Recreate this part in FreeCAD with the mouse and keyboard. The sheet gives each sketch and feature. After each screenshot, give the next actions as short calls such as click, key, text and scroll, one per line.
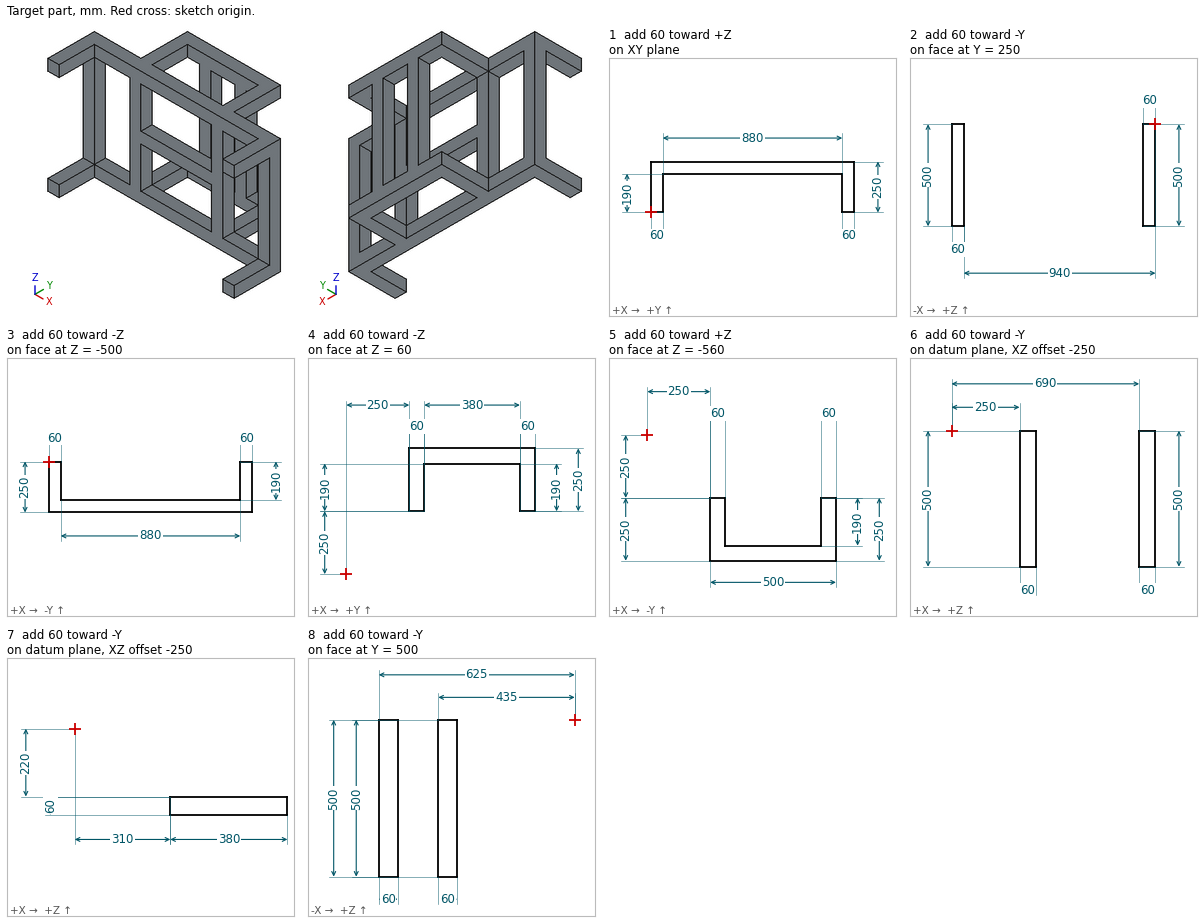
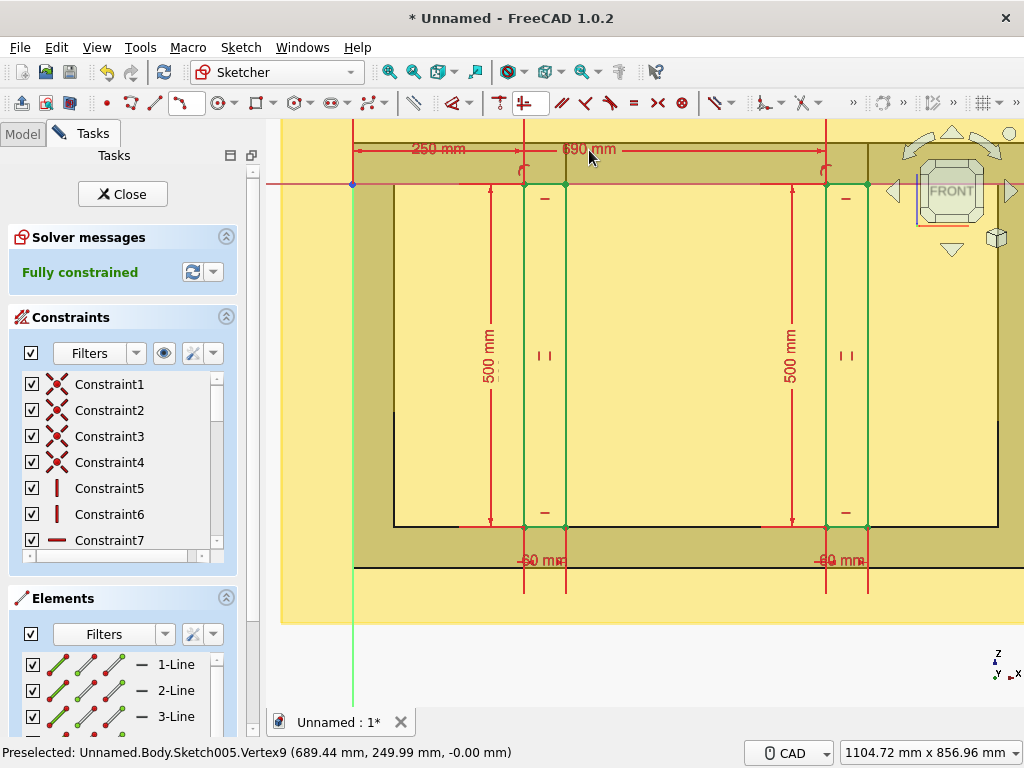
click(123, 194)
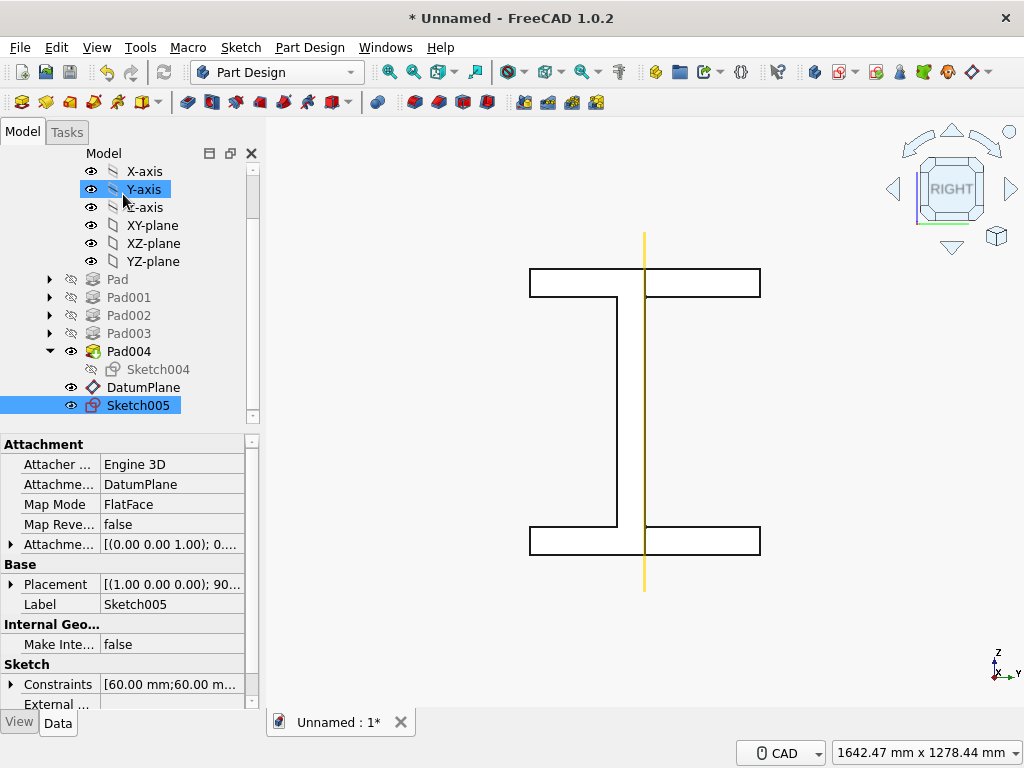
click(22, 102)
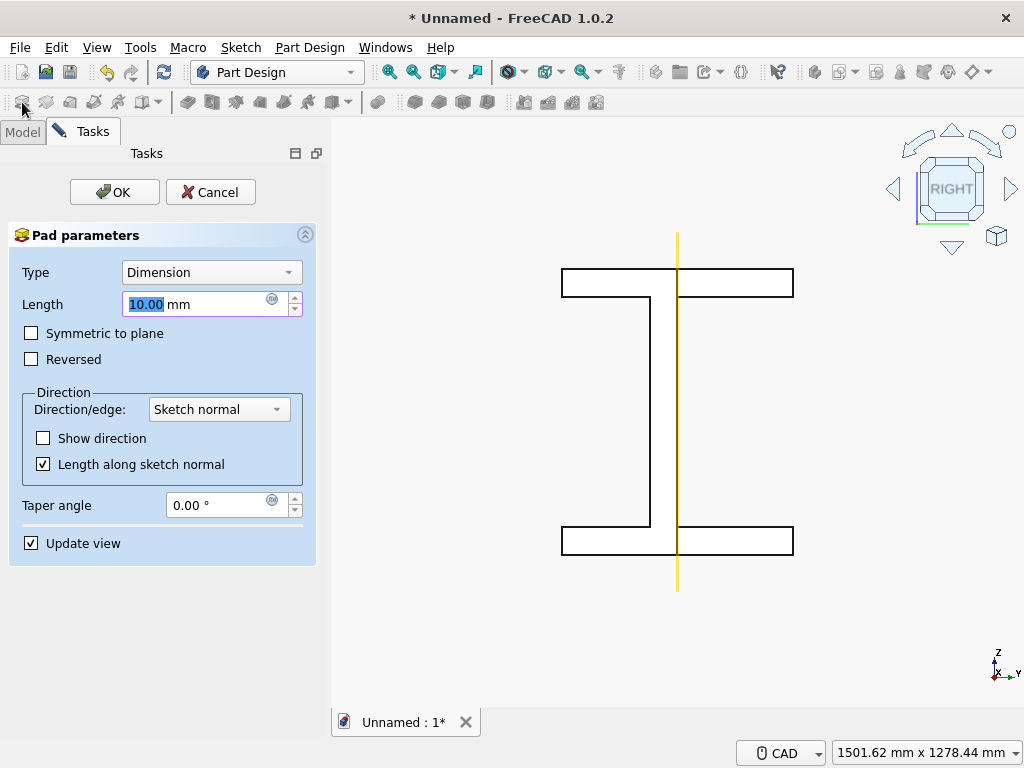
text(60)
key(Tab)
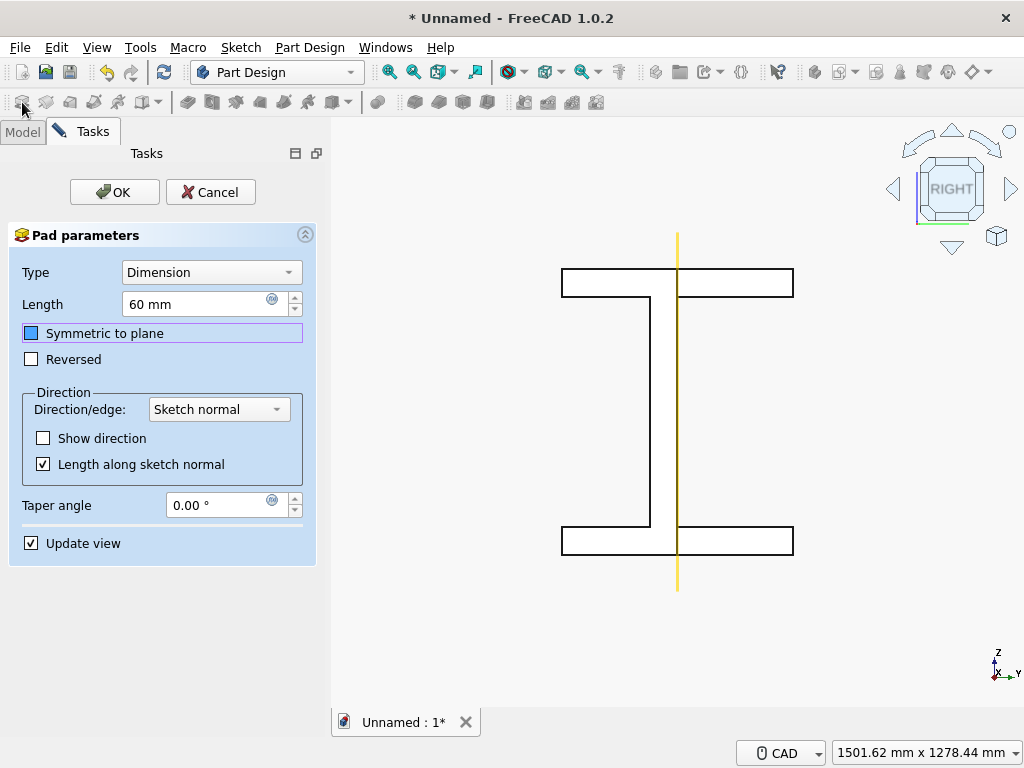
click(115, 192)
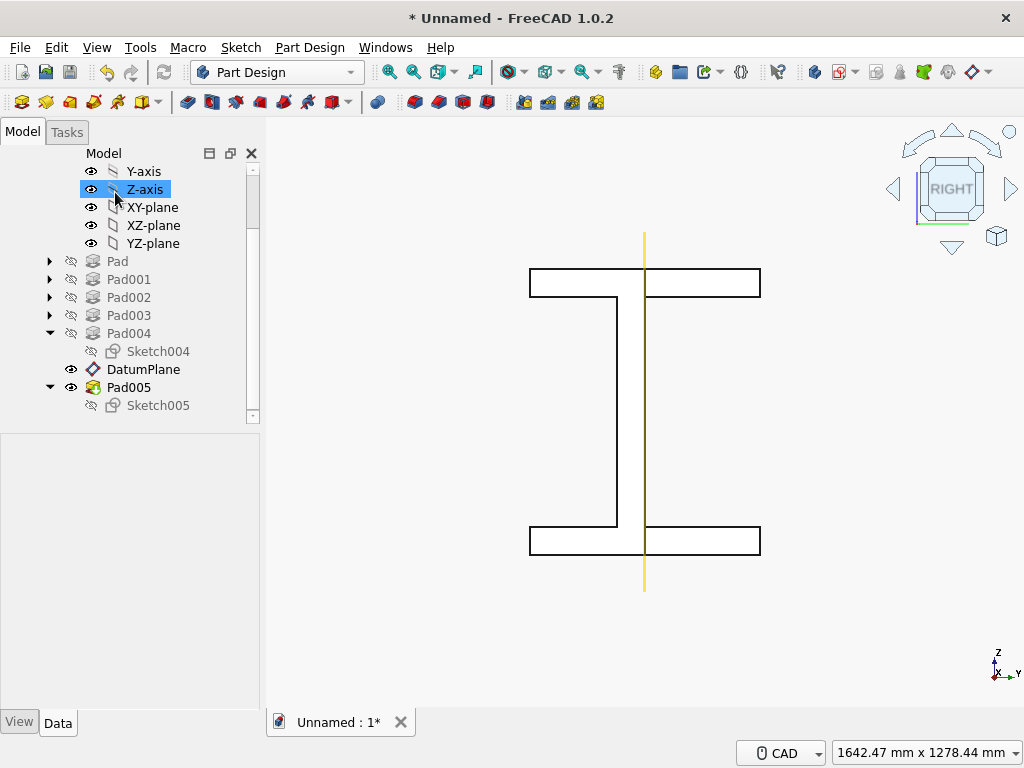
click(116, 369)
key(space)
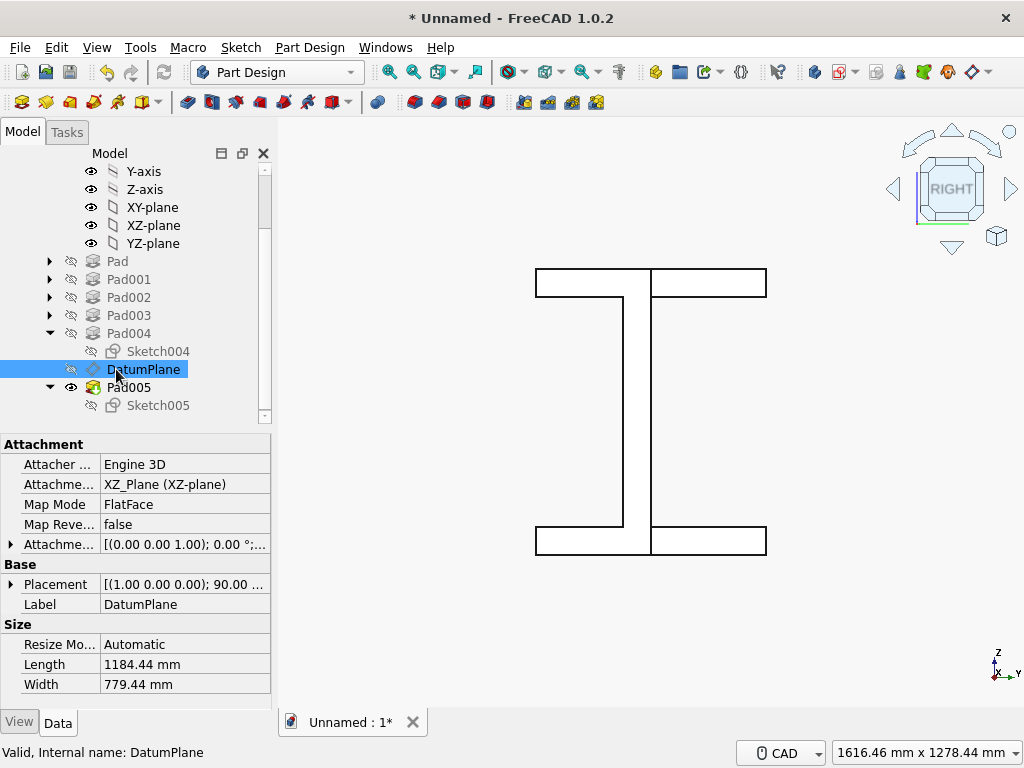
key(4)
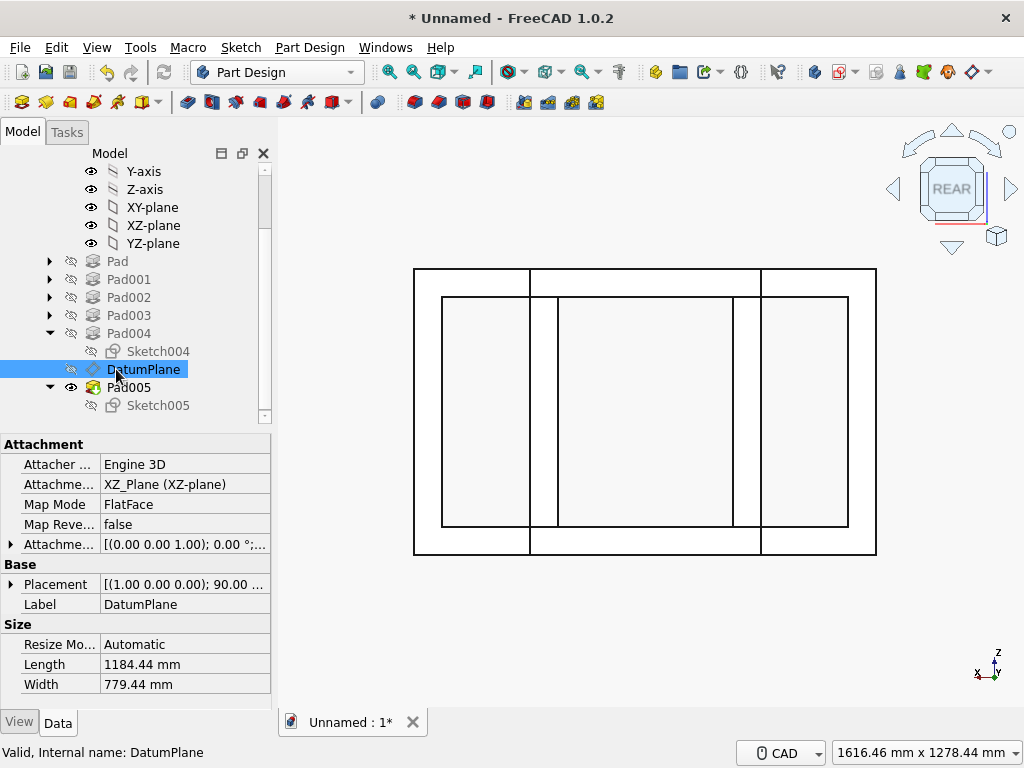
key(2)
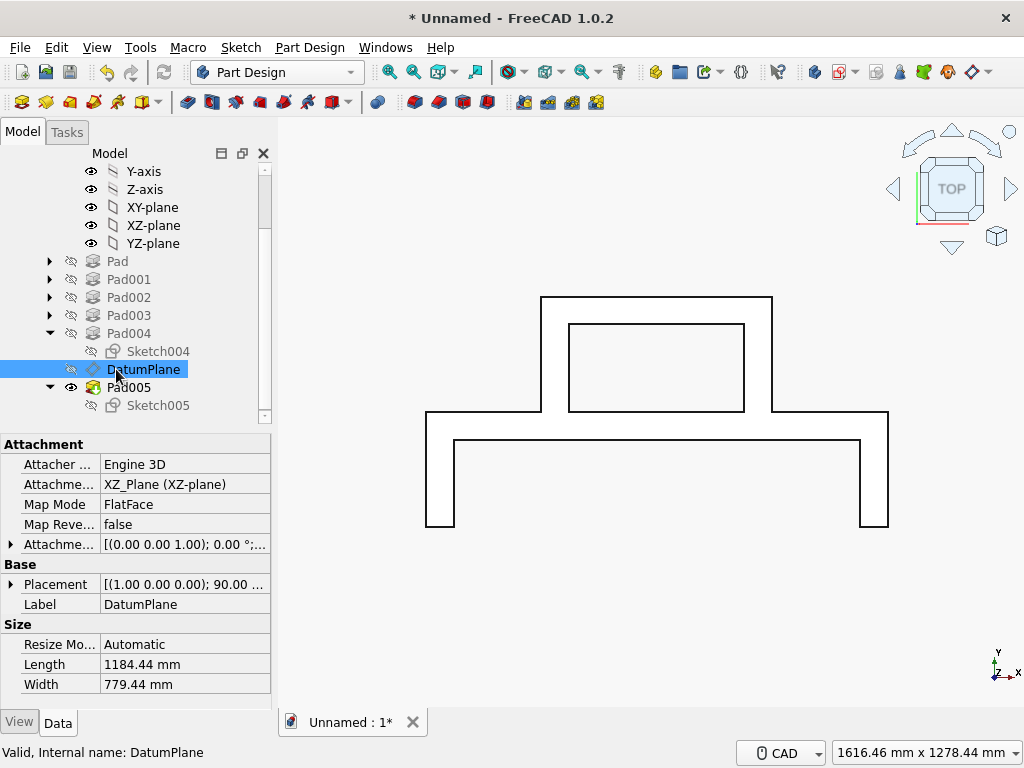
key(3)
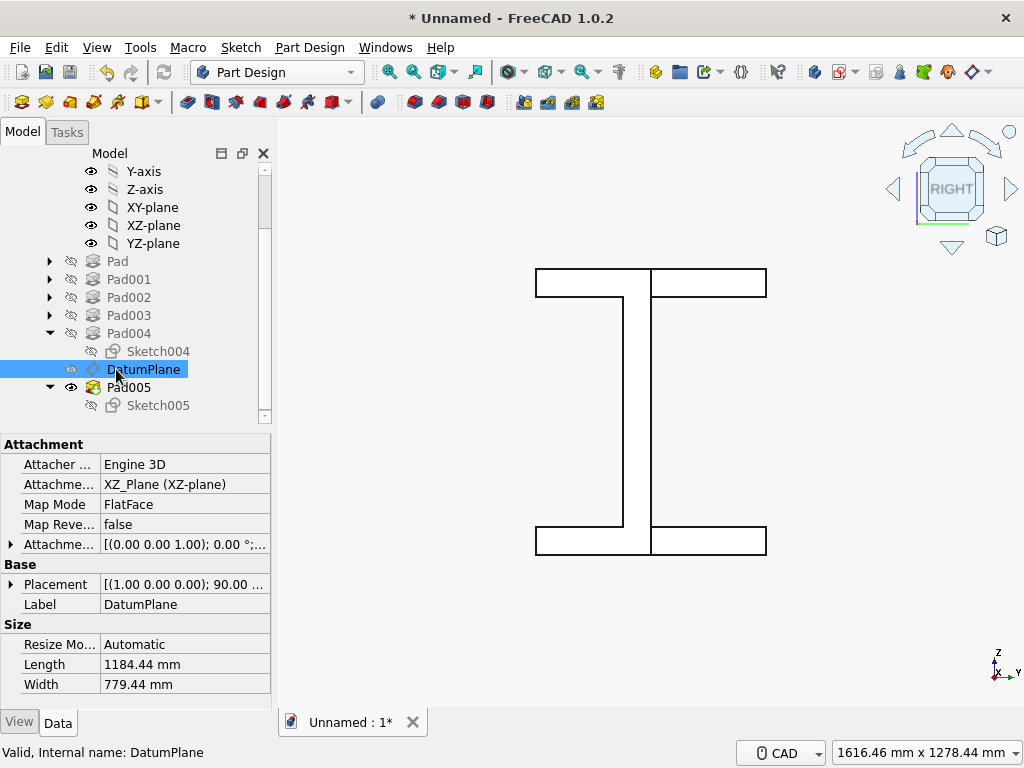
scroll(160, 293, down, 3)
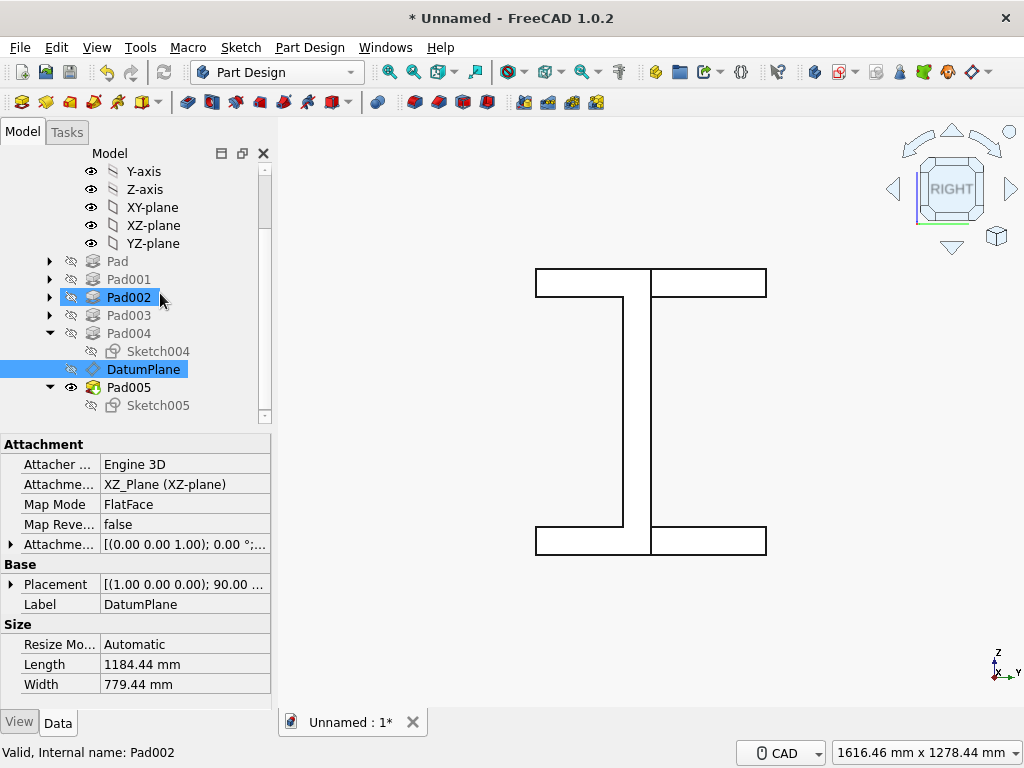
scroll(160, 293, up, 15)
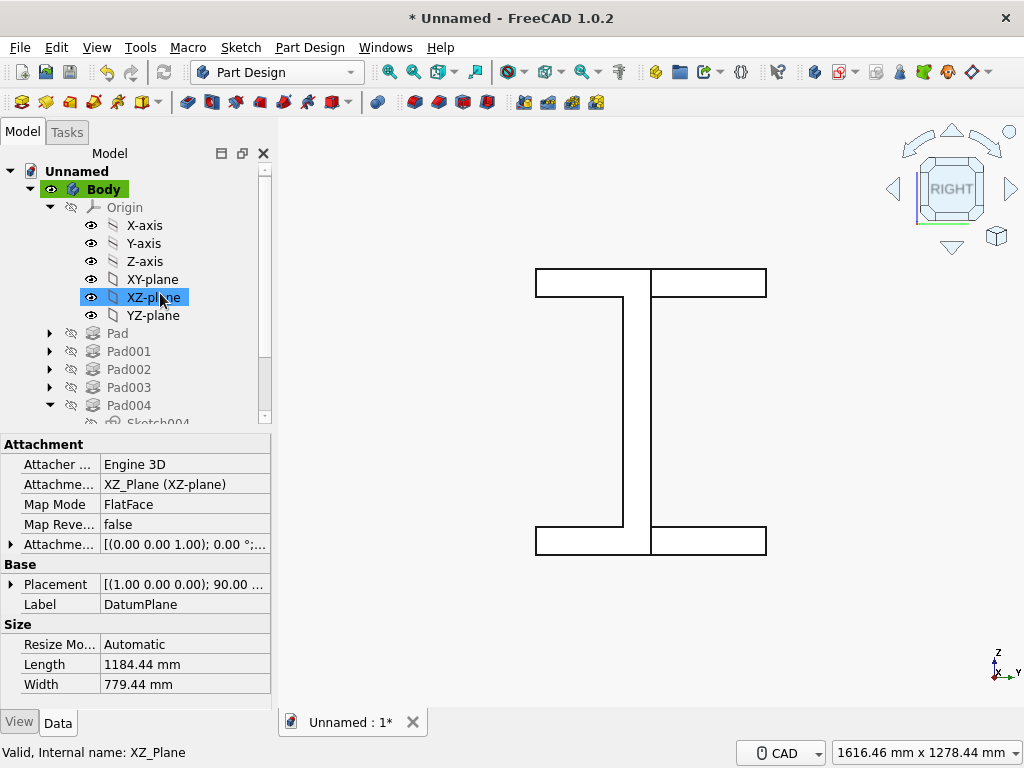
click(136, 297)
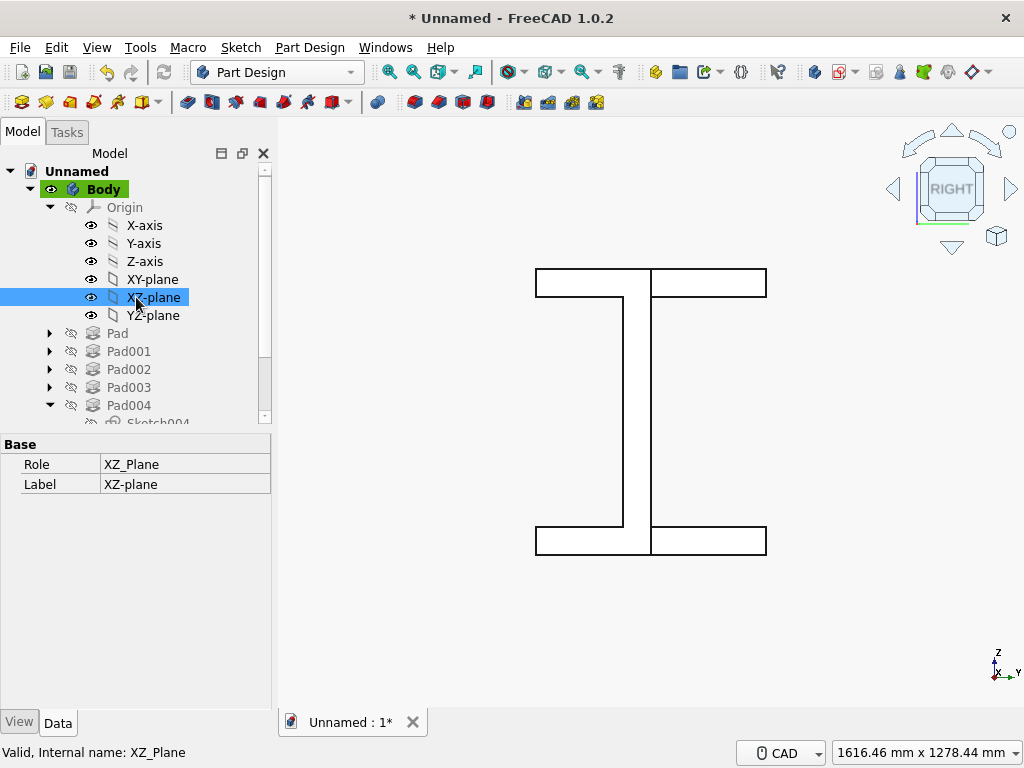
click(972, 72)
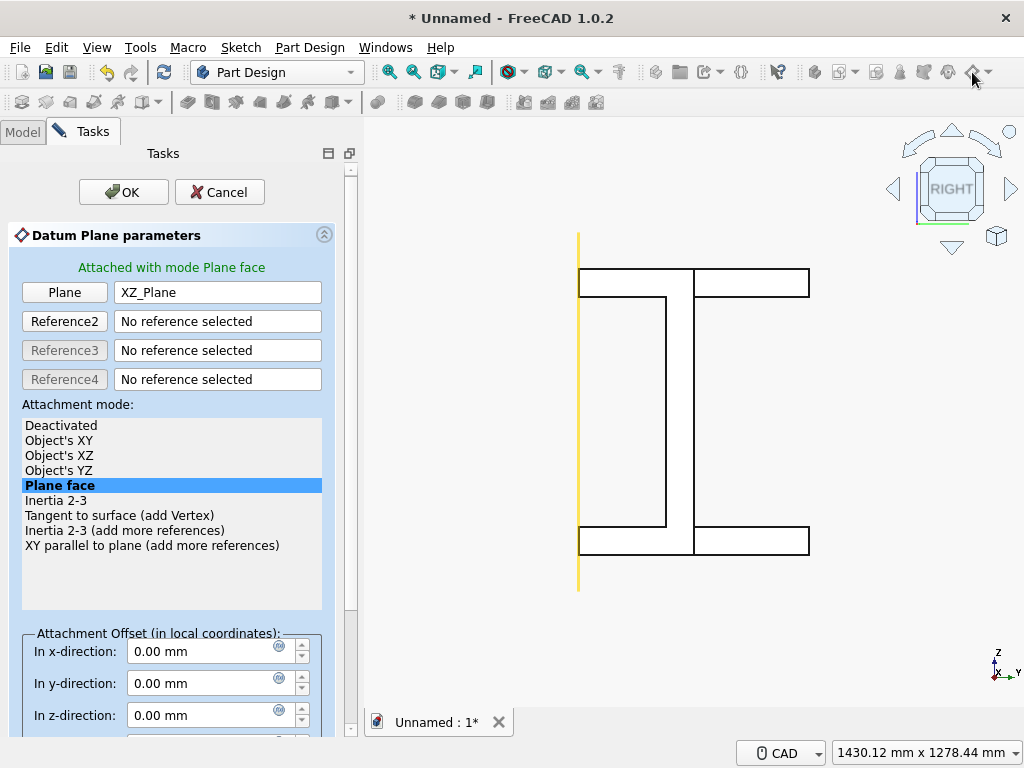
triple_click(210, 715)